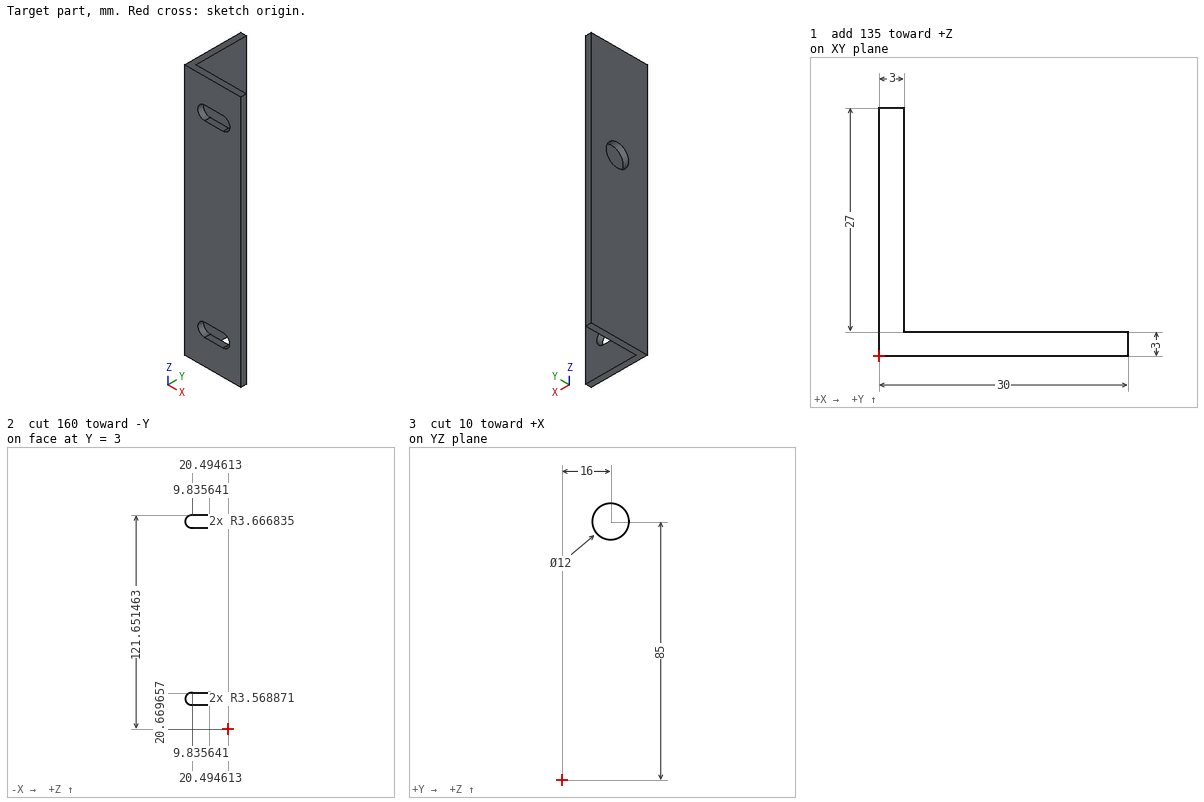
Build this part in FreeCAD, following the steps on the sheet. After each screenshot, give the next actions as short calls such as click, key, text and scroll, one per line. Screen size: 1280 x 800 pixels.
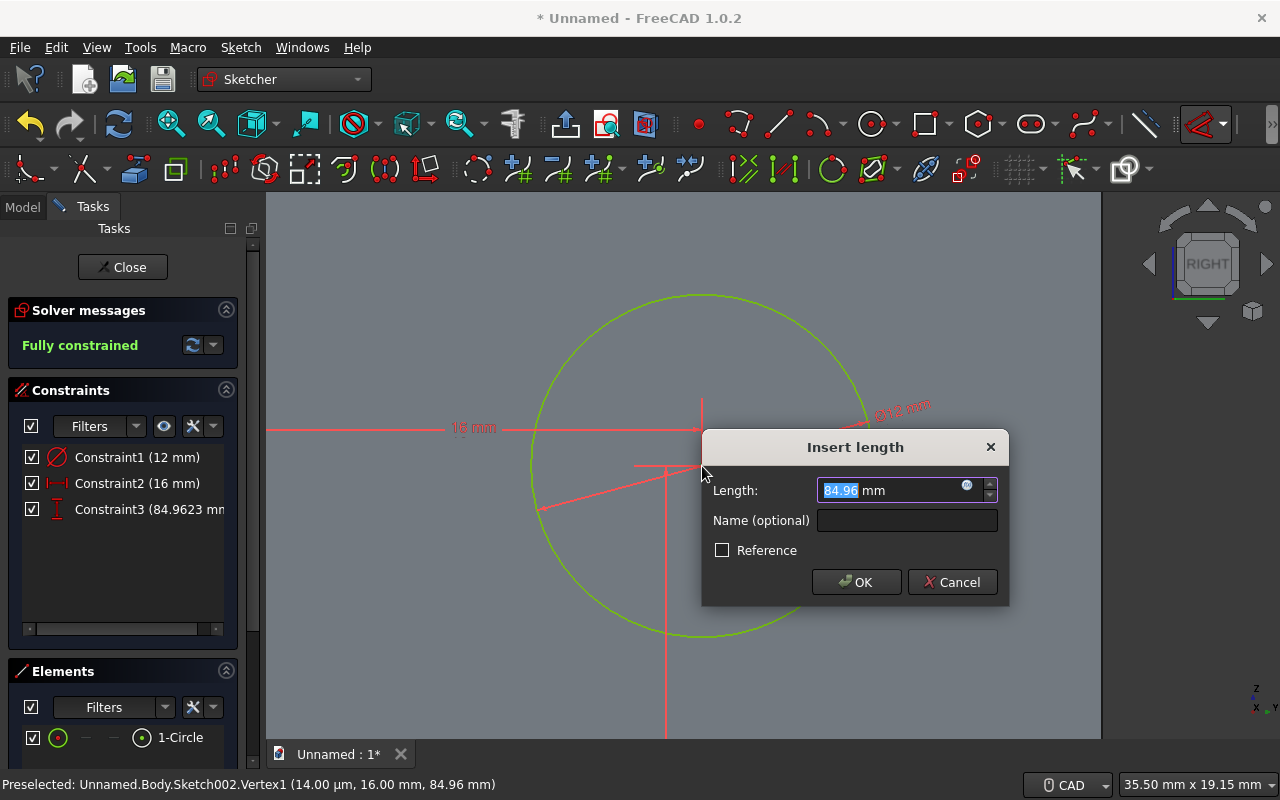
text(85)
key(Return)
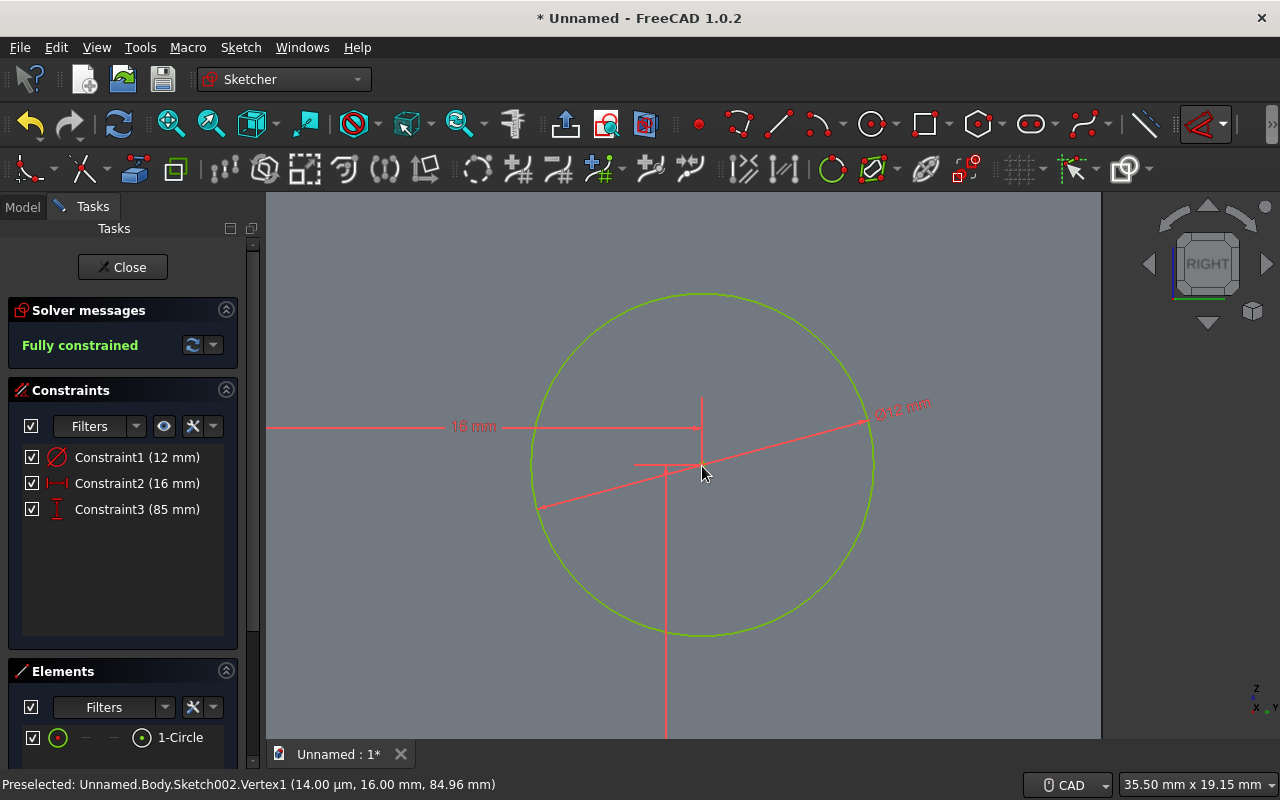
click(123, 267)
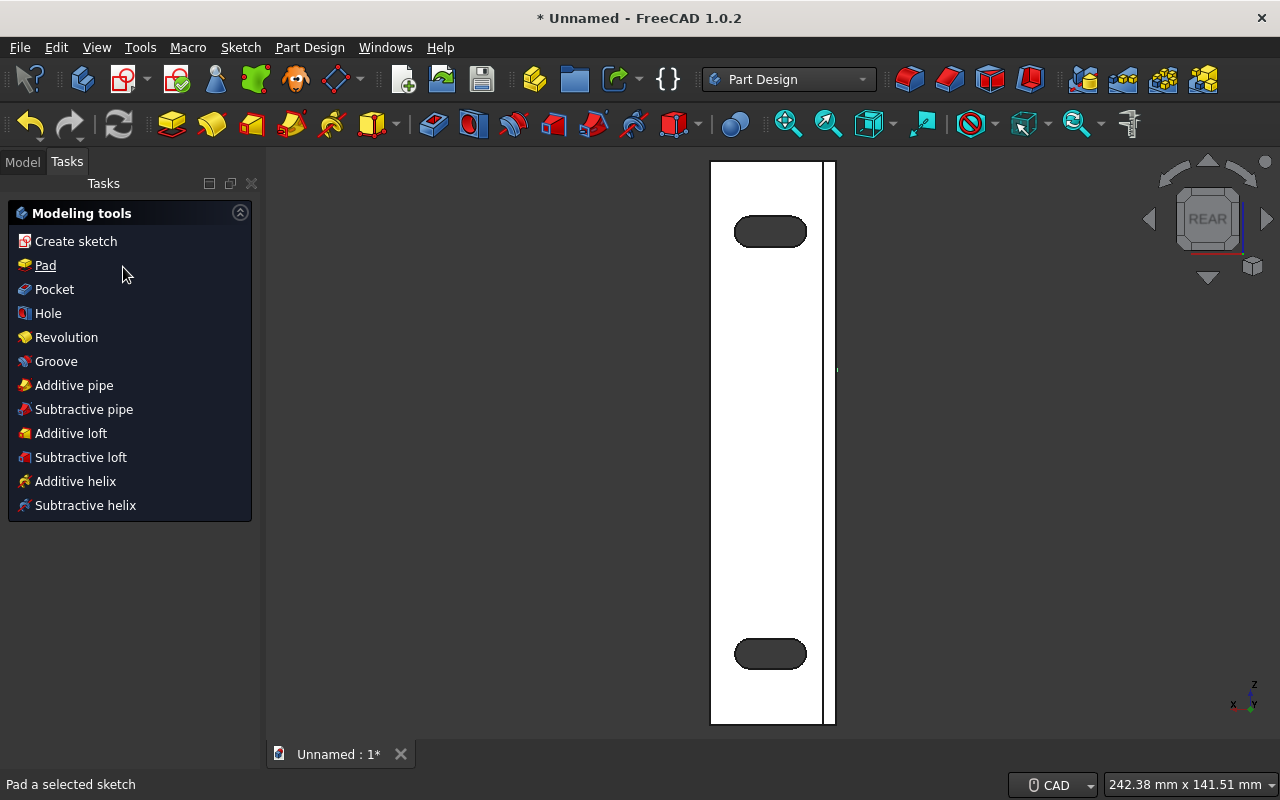
click(434, 124)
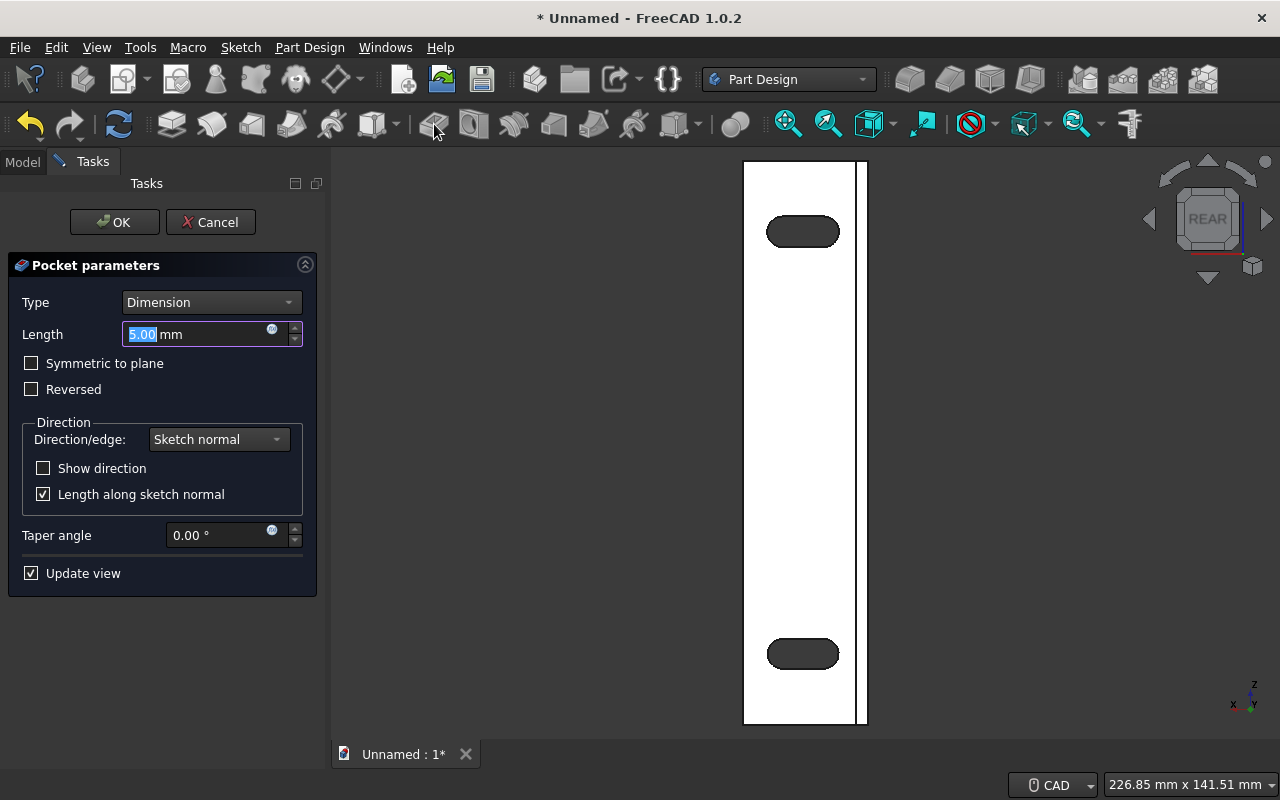
text(10)
key(Tab)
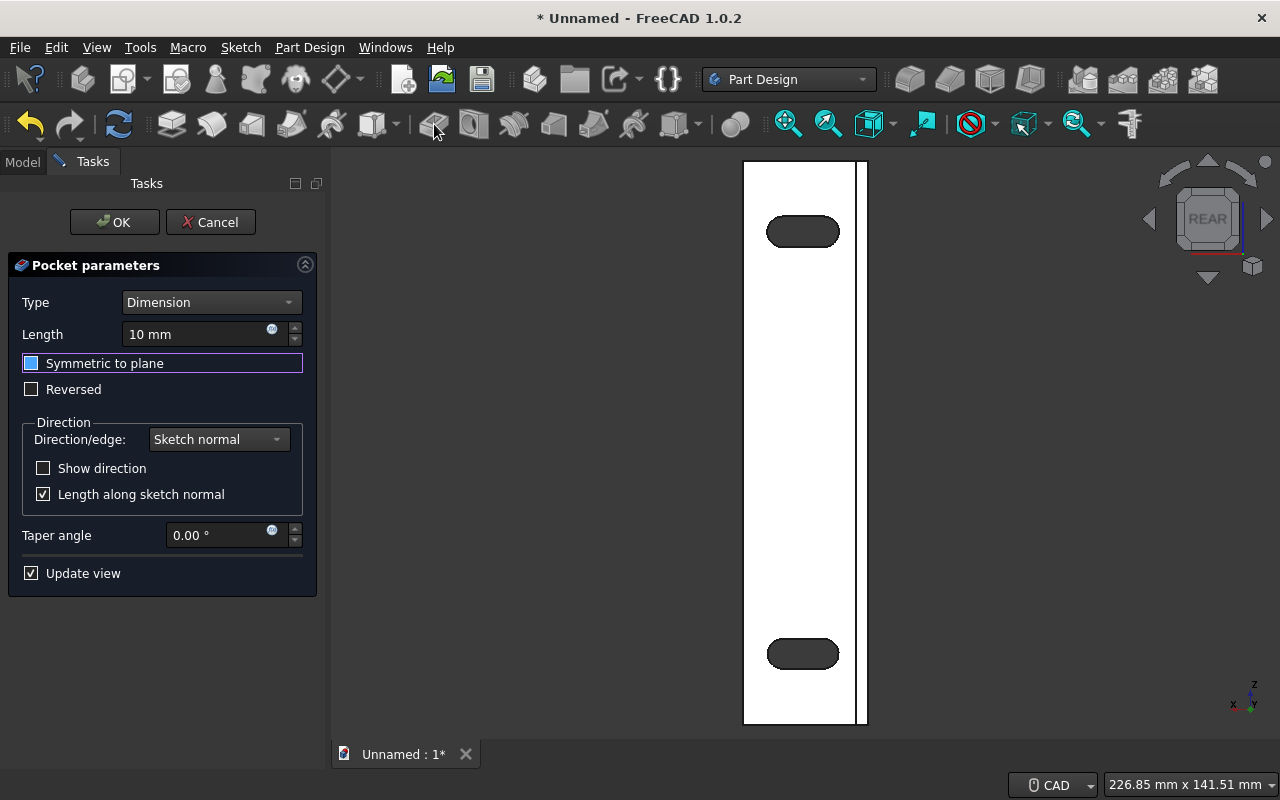
click(30, 389)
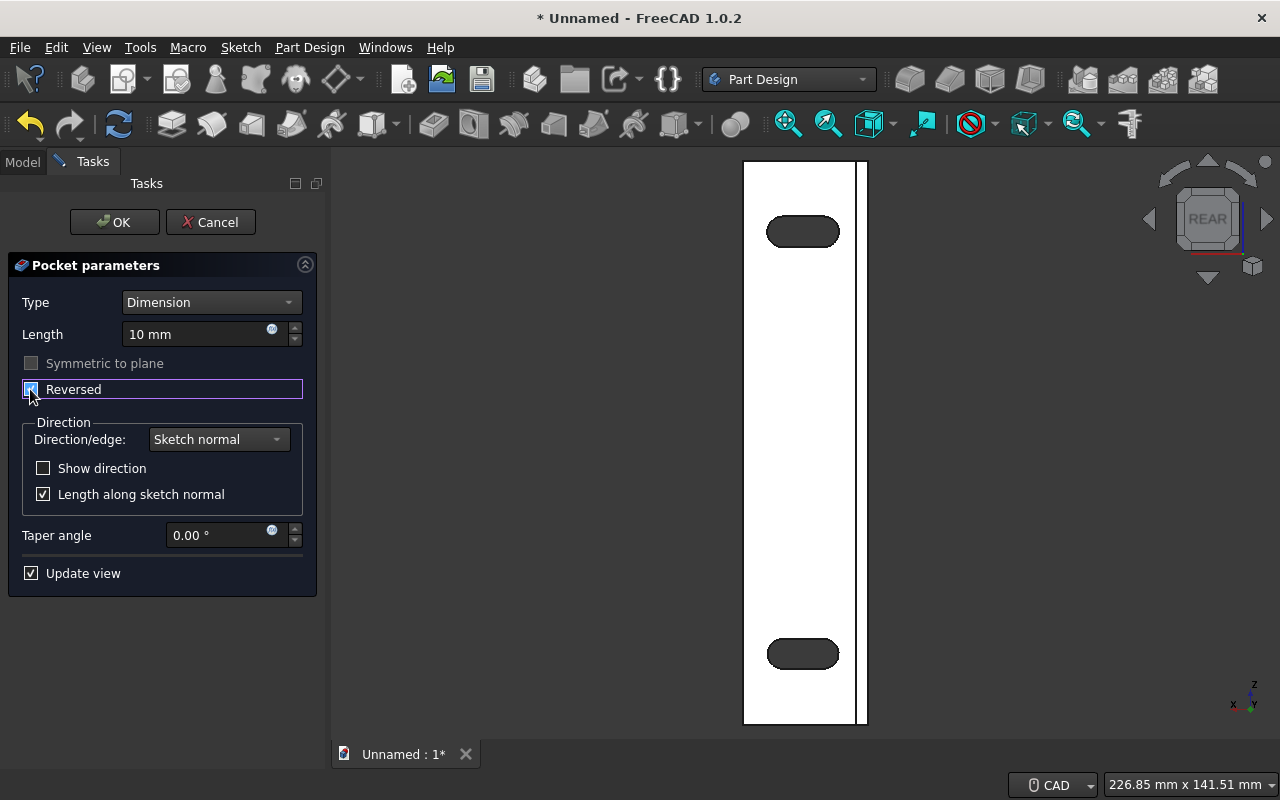
click(115, 222)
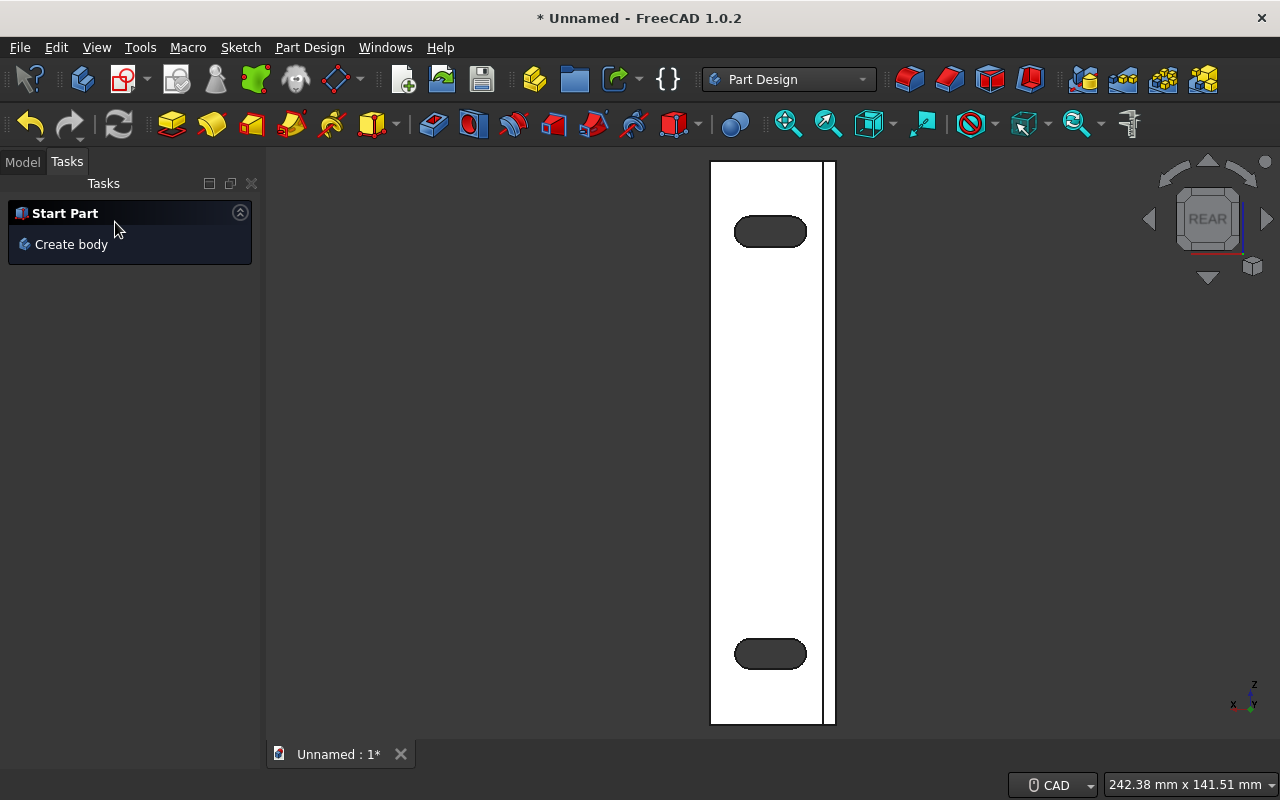
key(0)